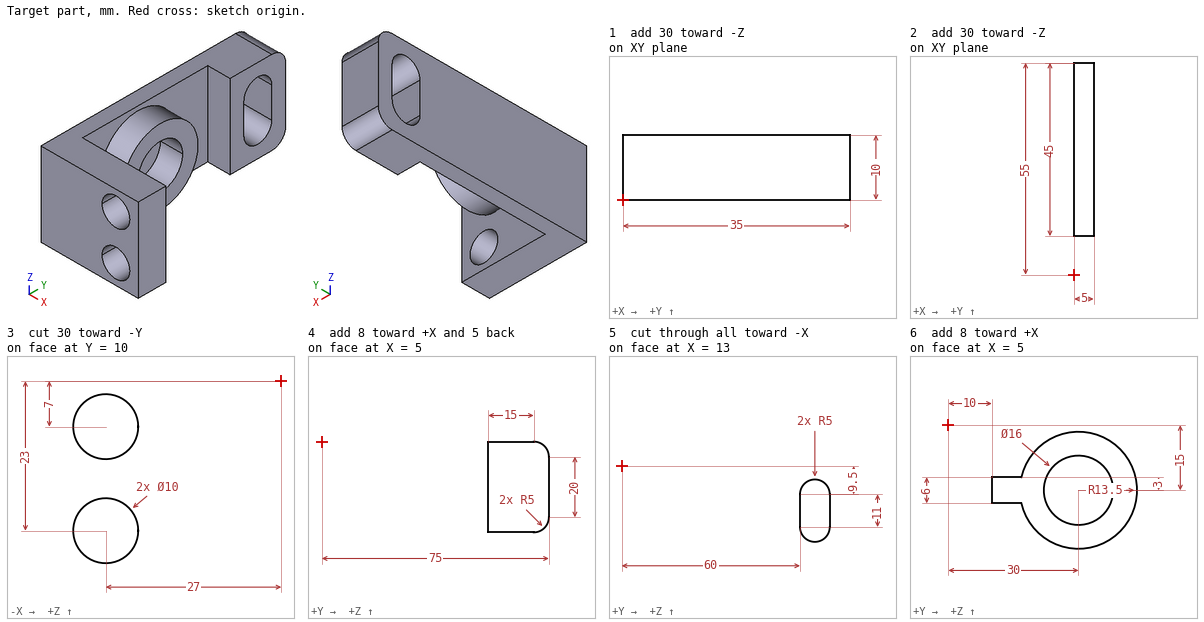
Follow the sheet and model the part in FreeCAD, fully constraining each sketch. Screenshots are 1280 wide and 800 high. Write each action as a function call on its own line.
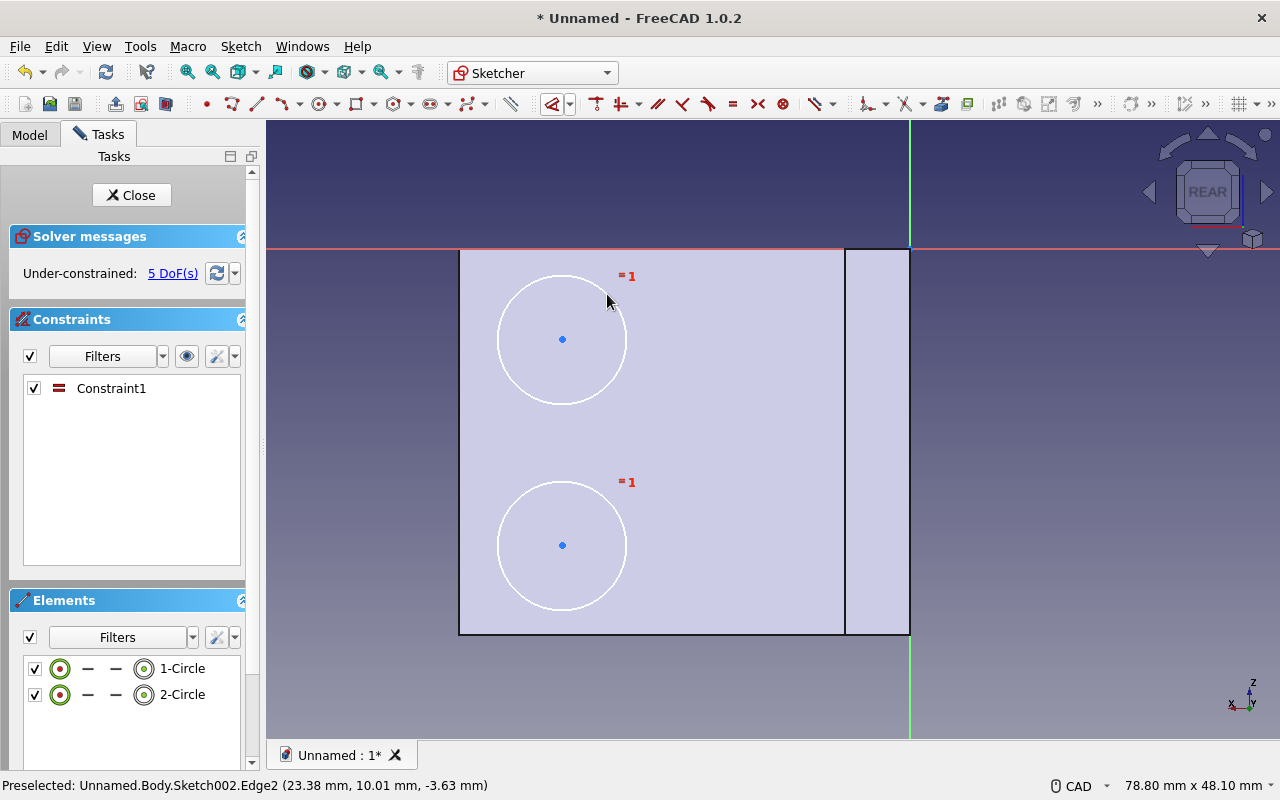
click(562, 546)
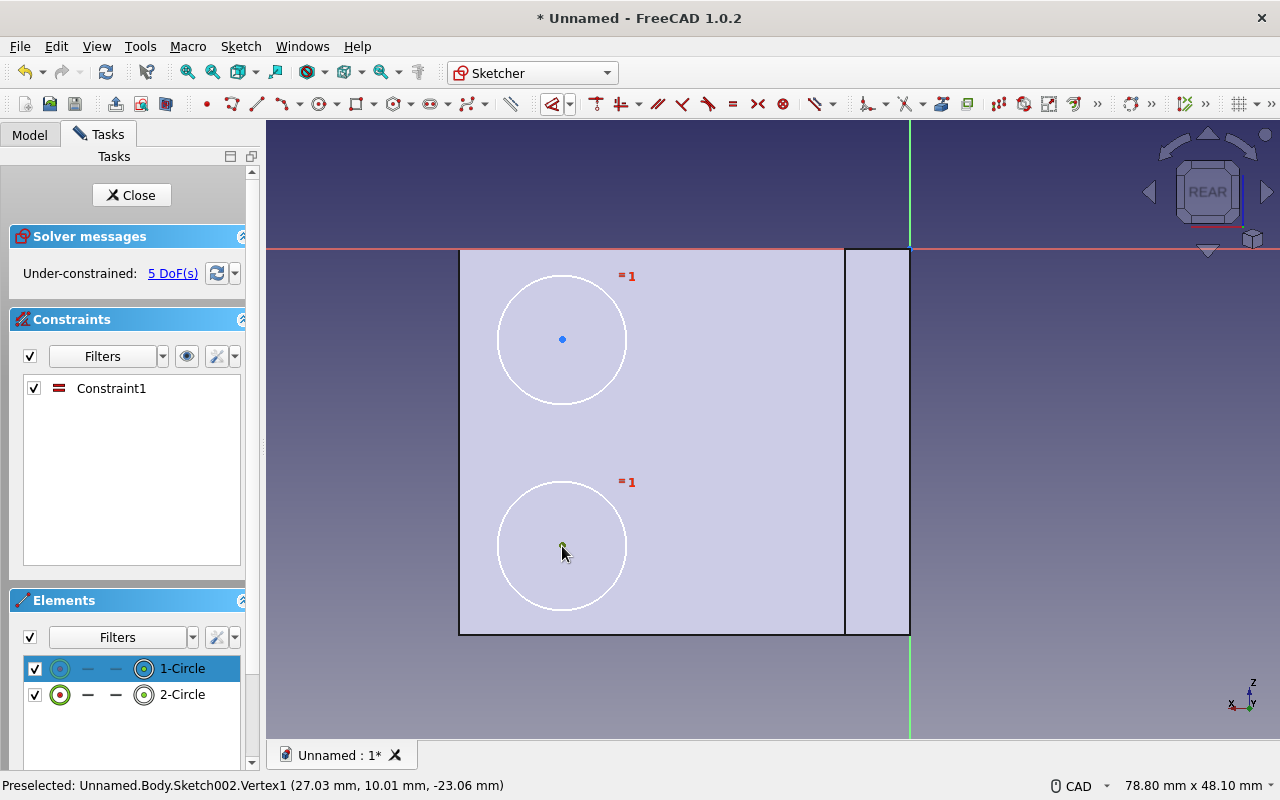
click(562, 340)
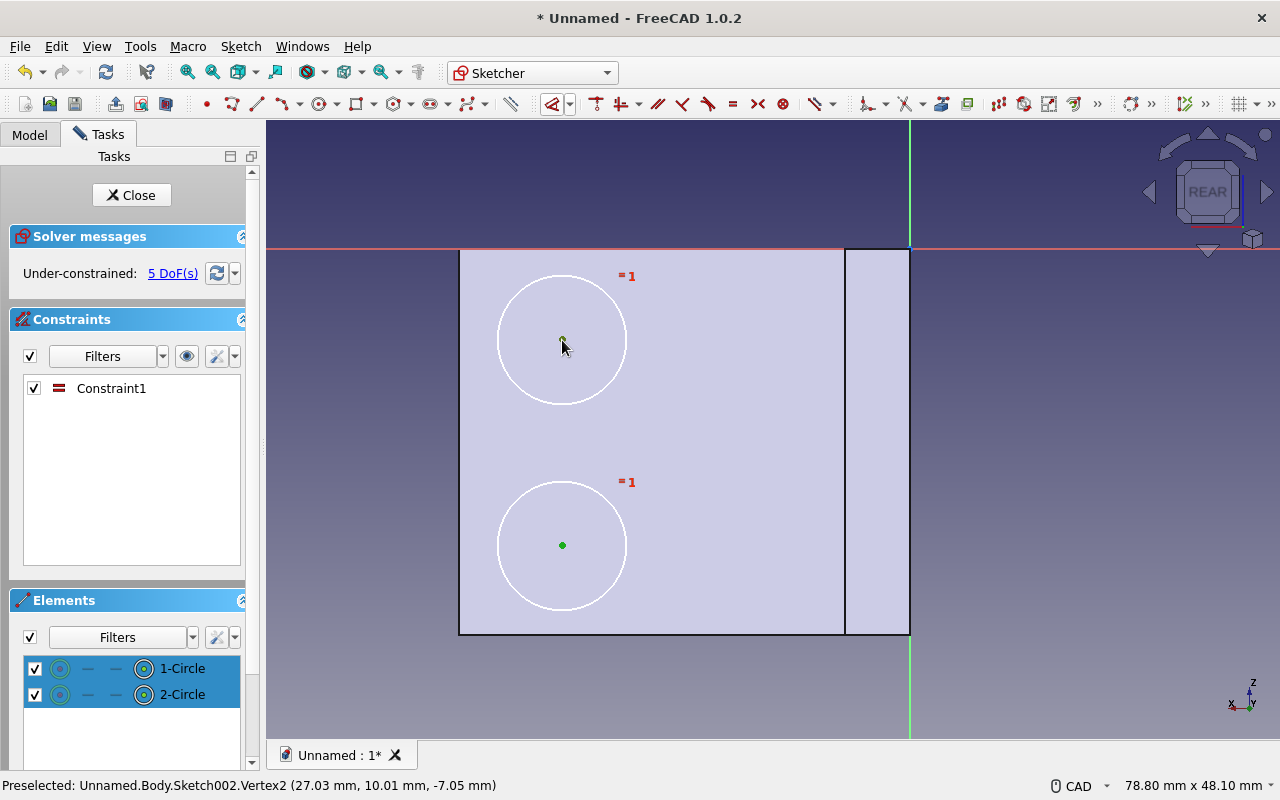
key(v)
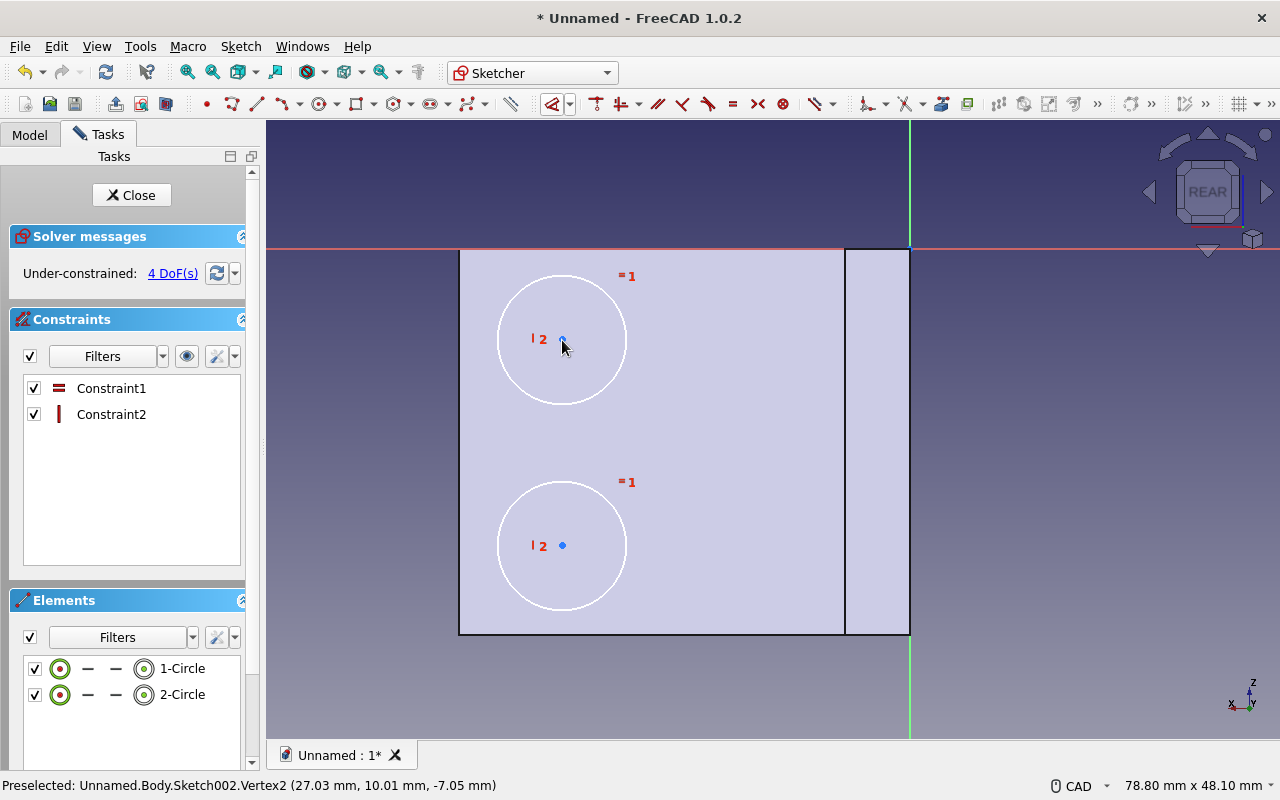
key(d)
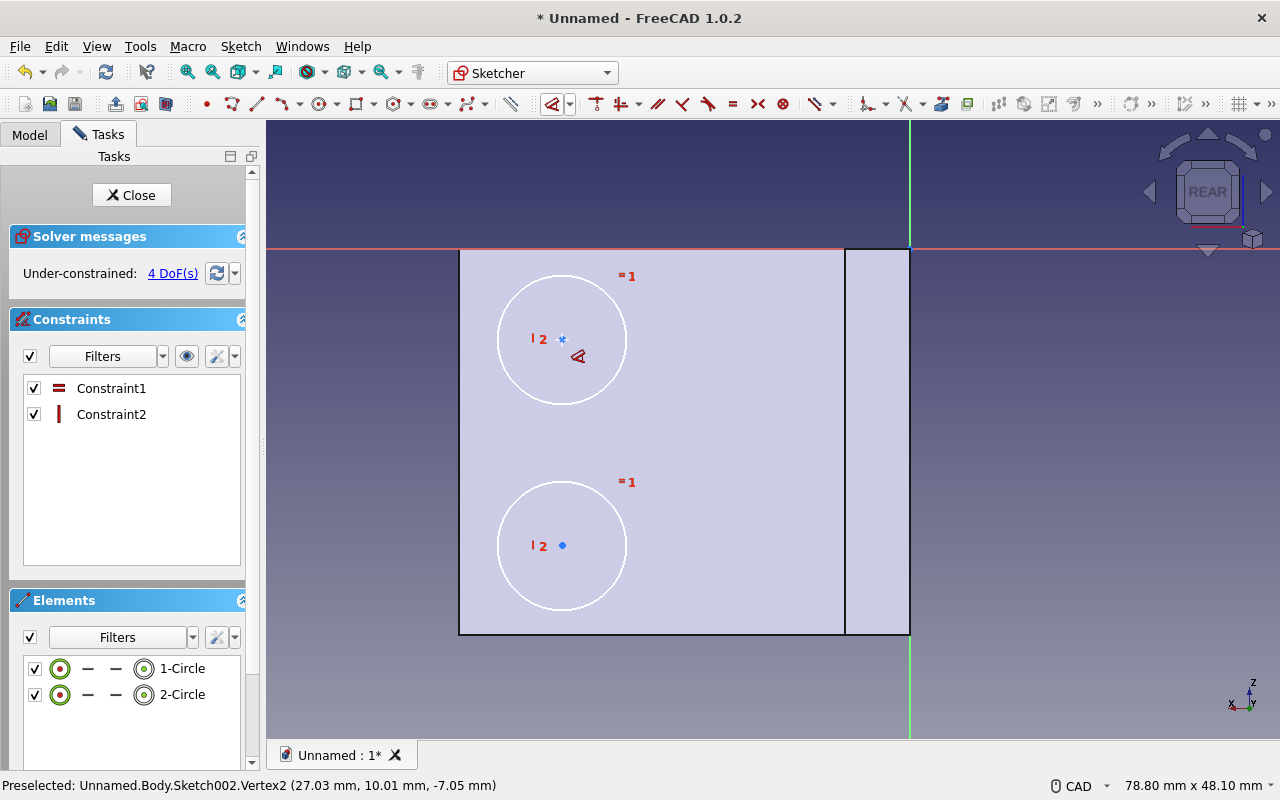
click(607, 500)
click(629, 477)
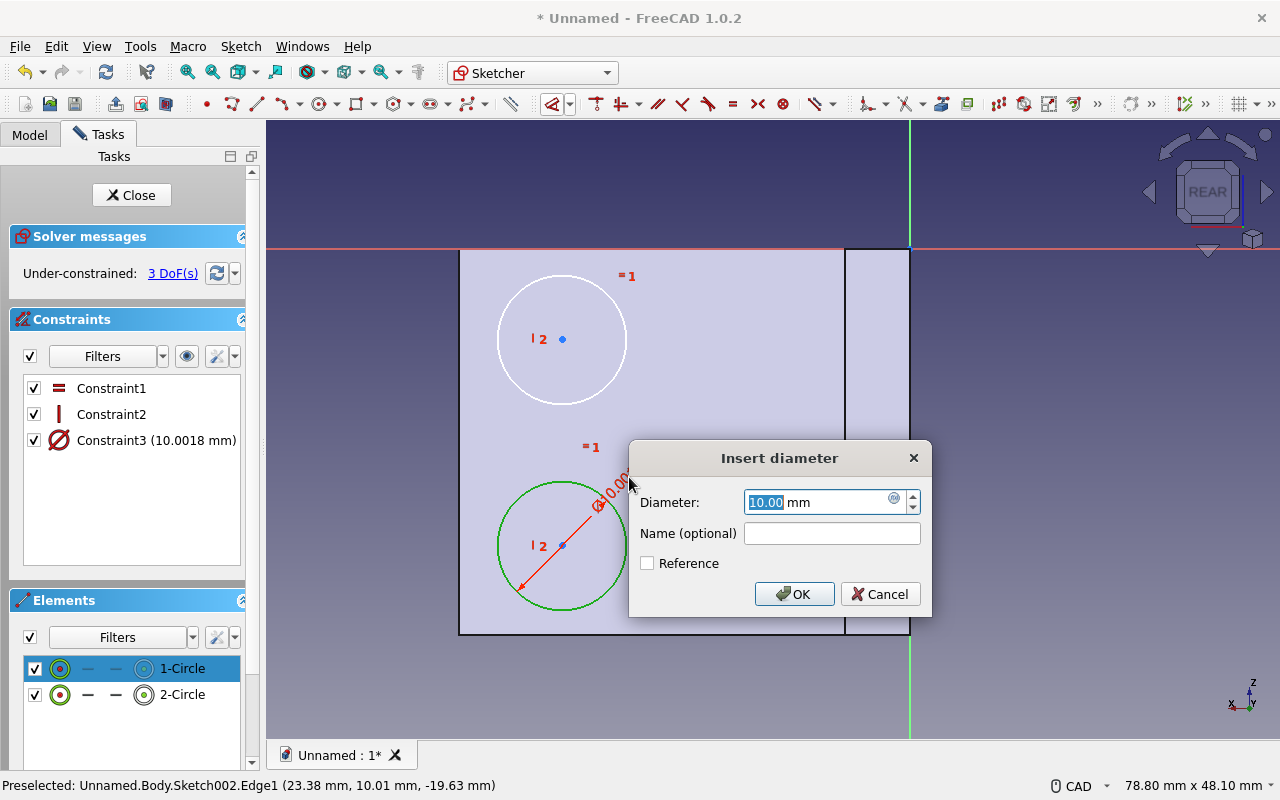
text(10)
key(Return)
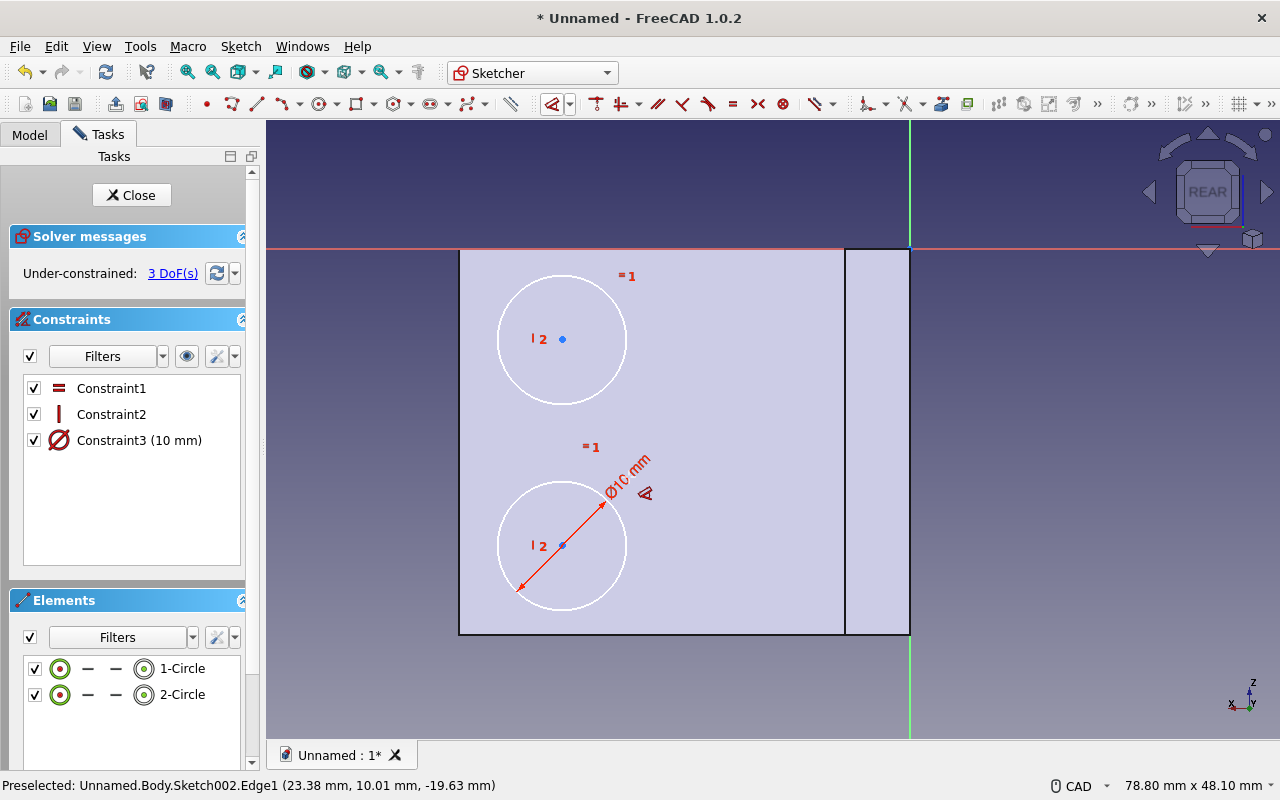
click(562, 340)
click(944, 295)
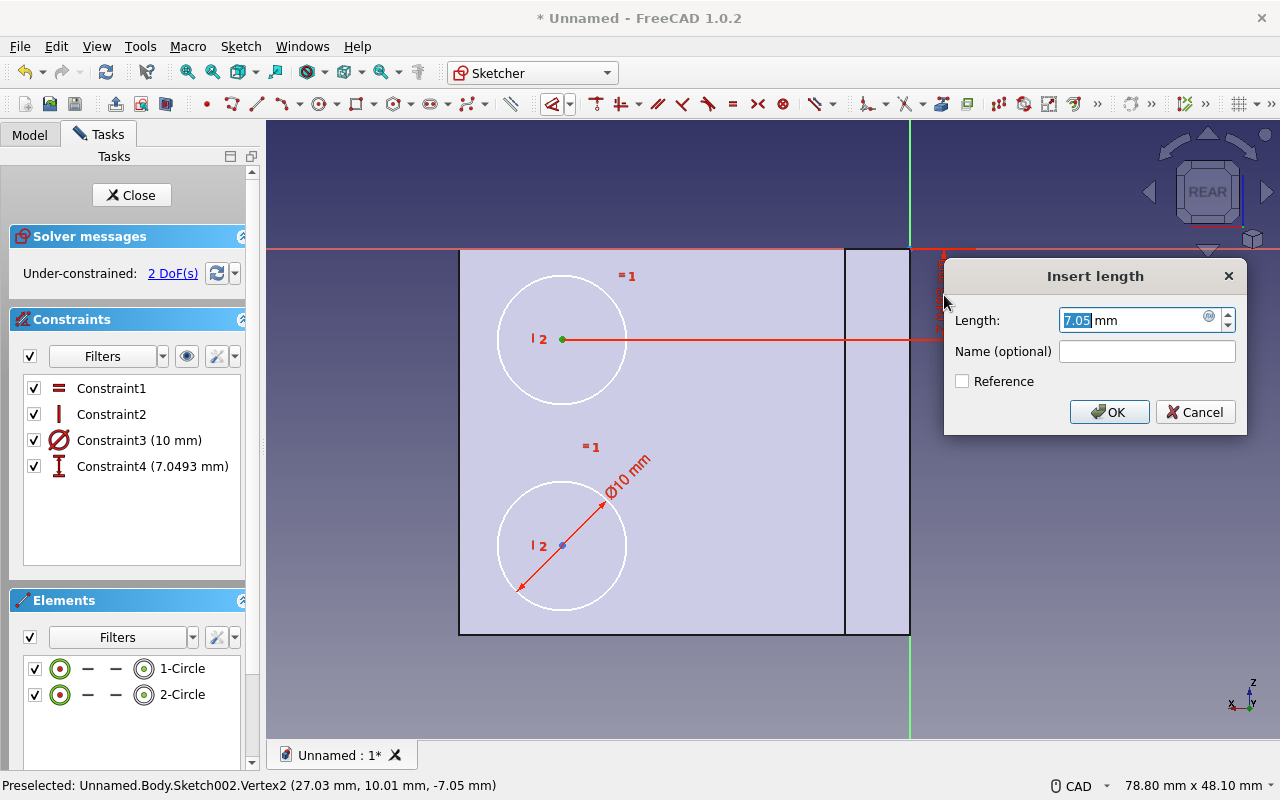
text(7)
key(Return)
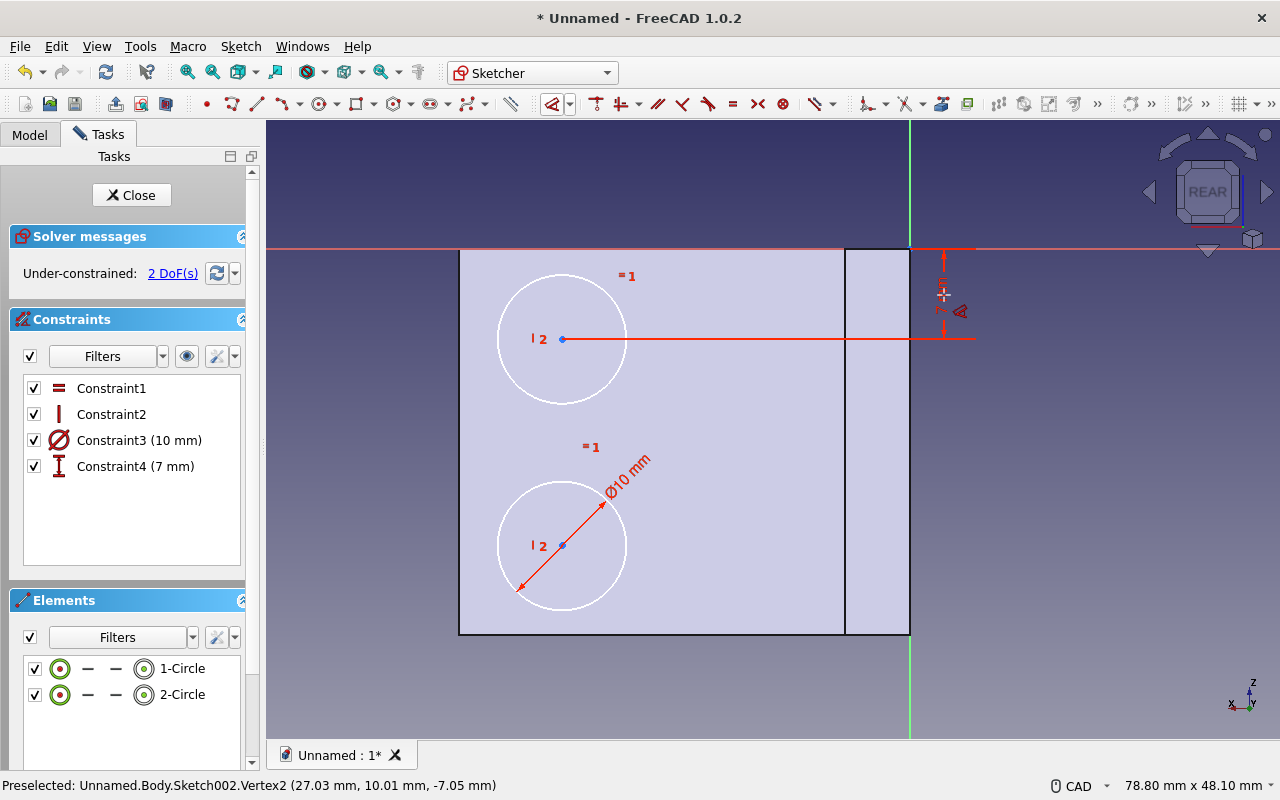
click(562, 546)
click(736, 215)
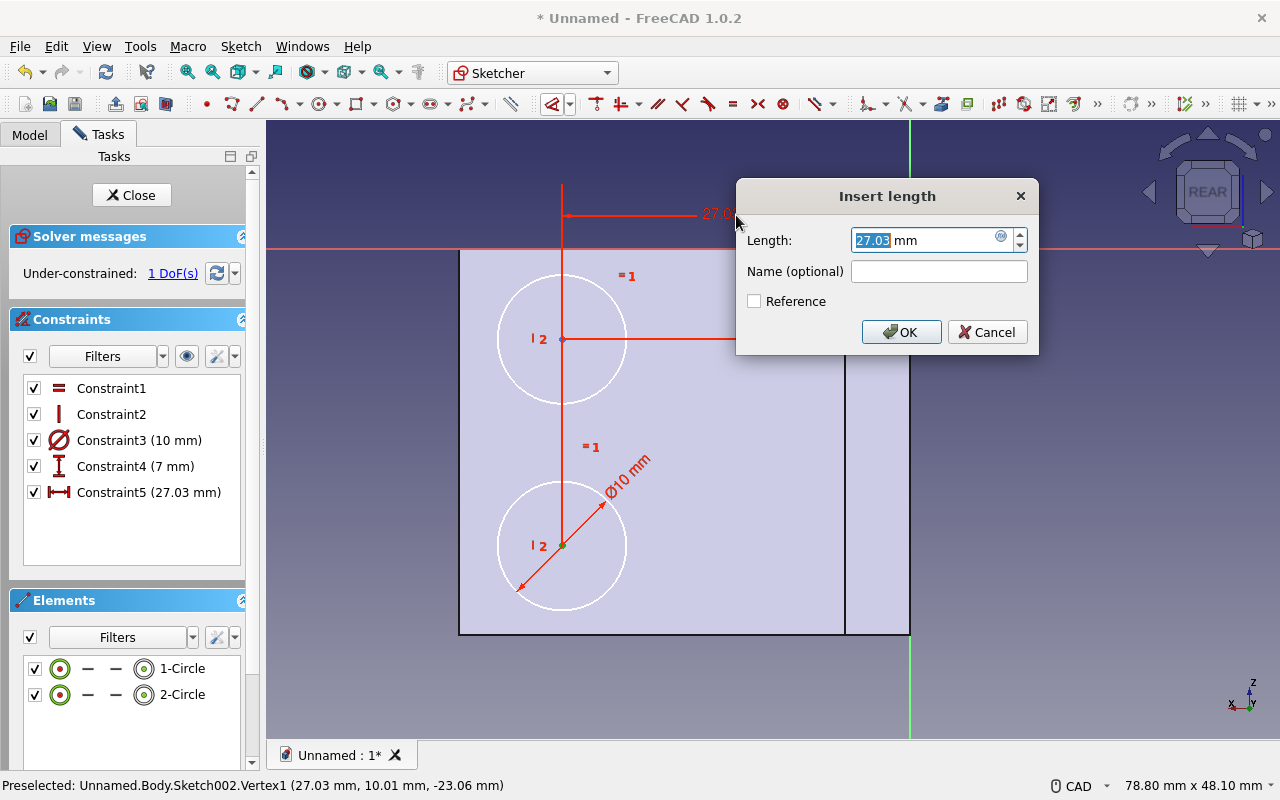
text(27)
key(Return)